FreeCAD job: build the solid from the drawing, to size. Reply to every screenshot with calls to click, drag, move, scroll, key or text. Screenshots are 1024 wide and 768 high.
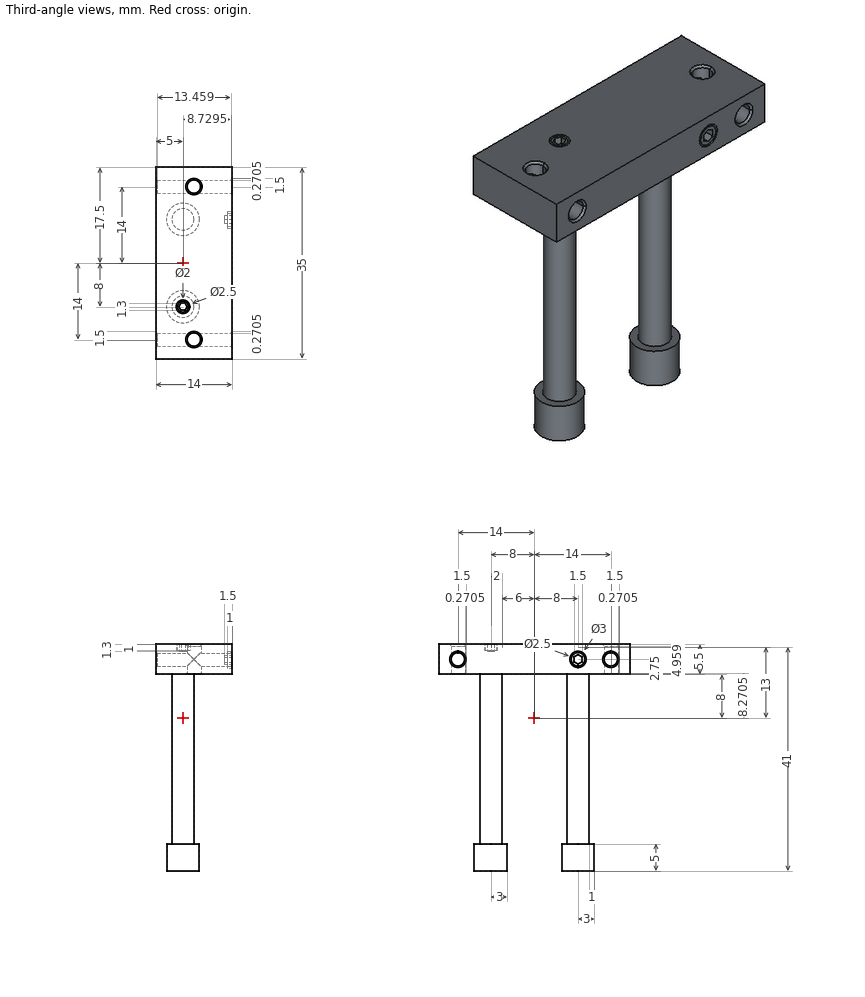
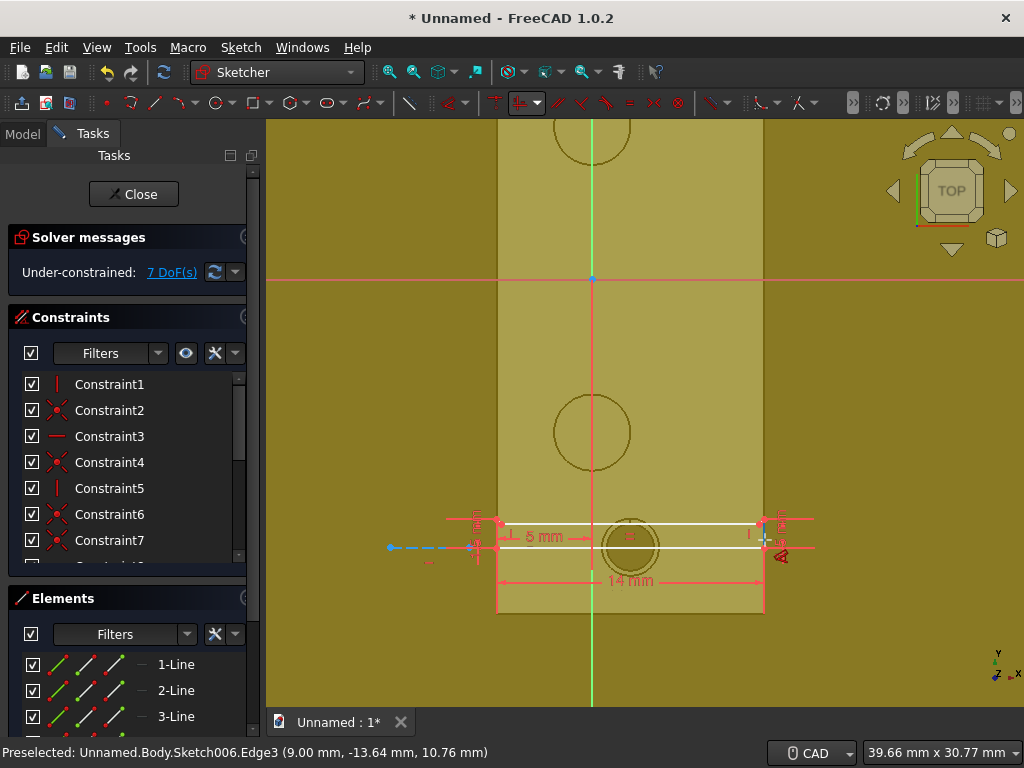
click(497, 548)
click(463, 414)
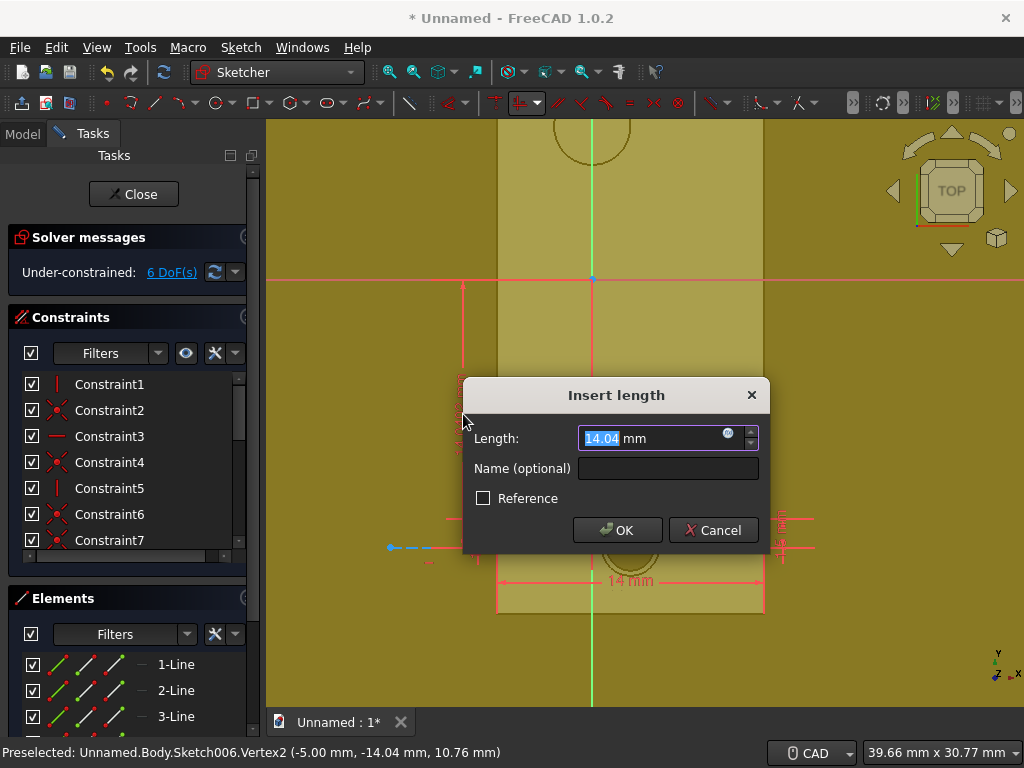
text(14)
key(Return)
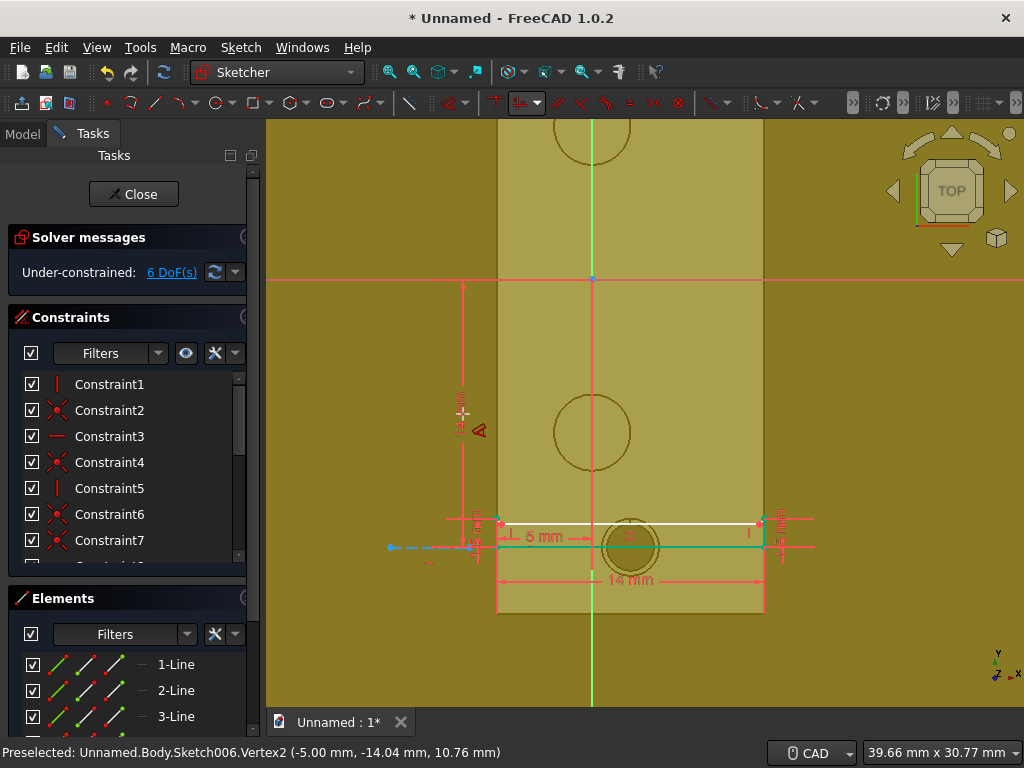
click(470, 548)
click(436, 352)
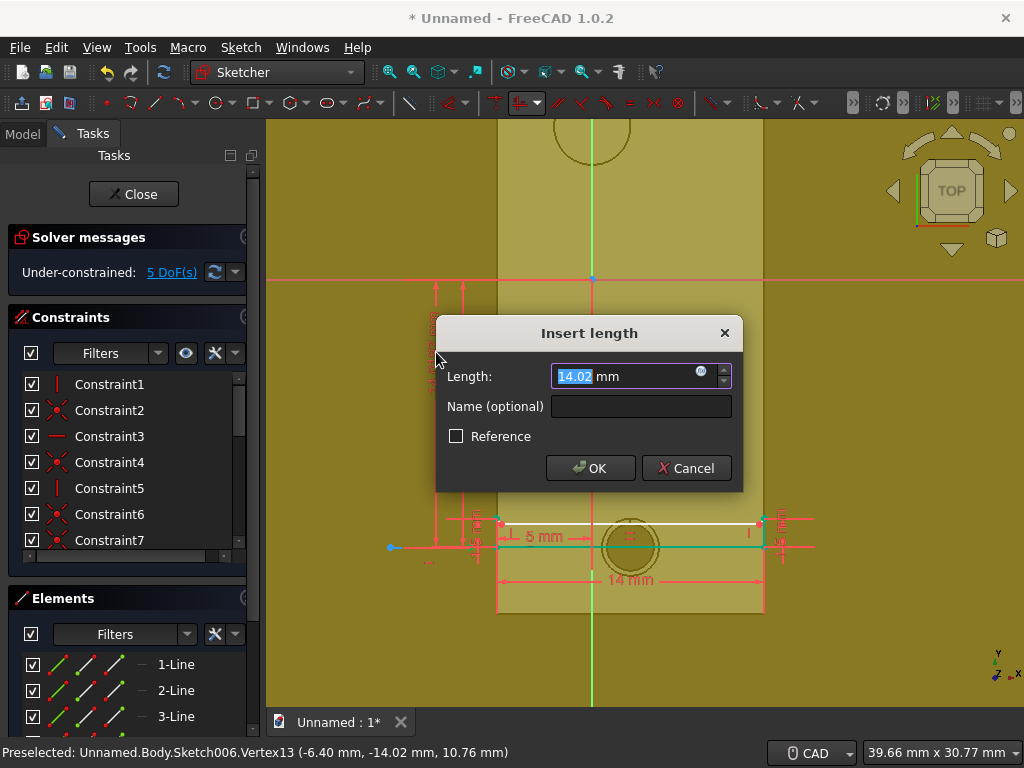
text(14)
key(Return)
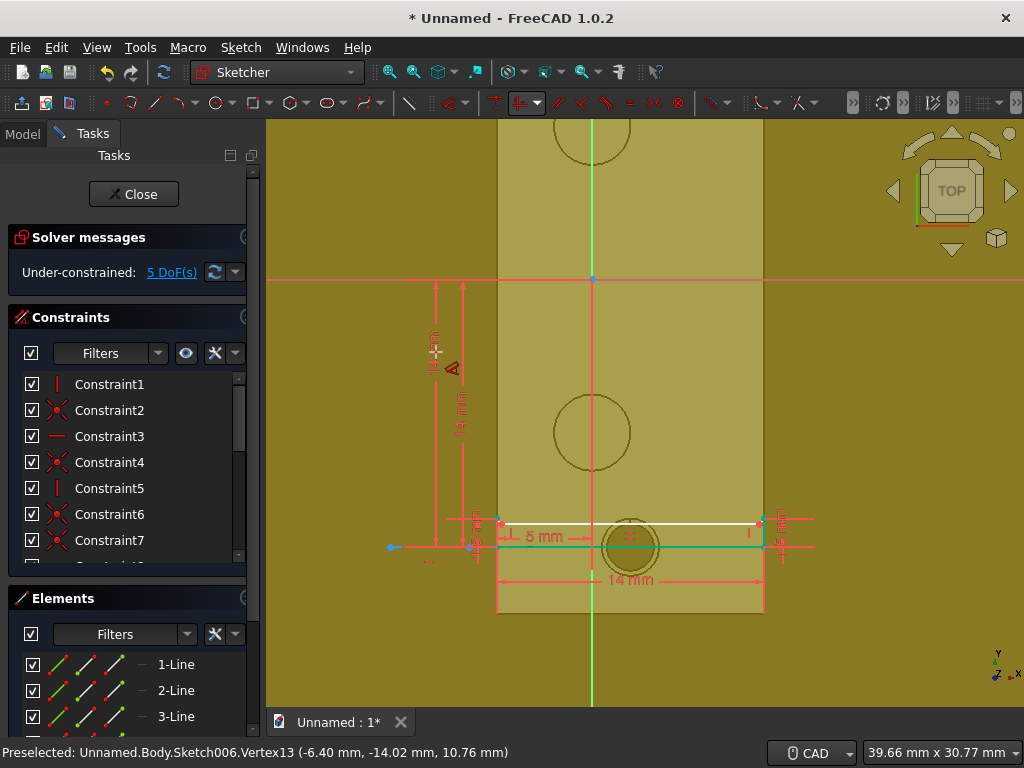
click(682, 524)
click(631, 490)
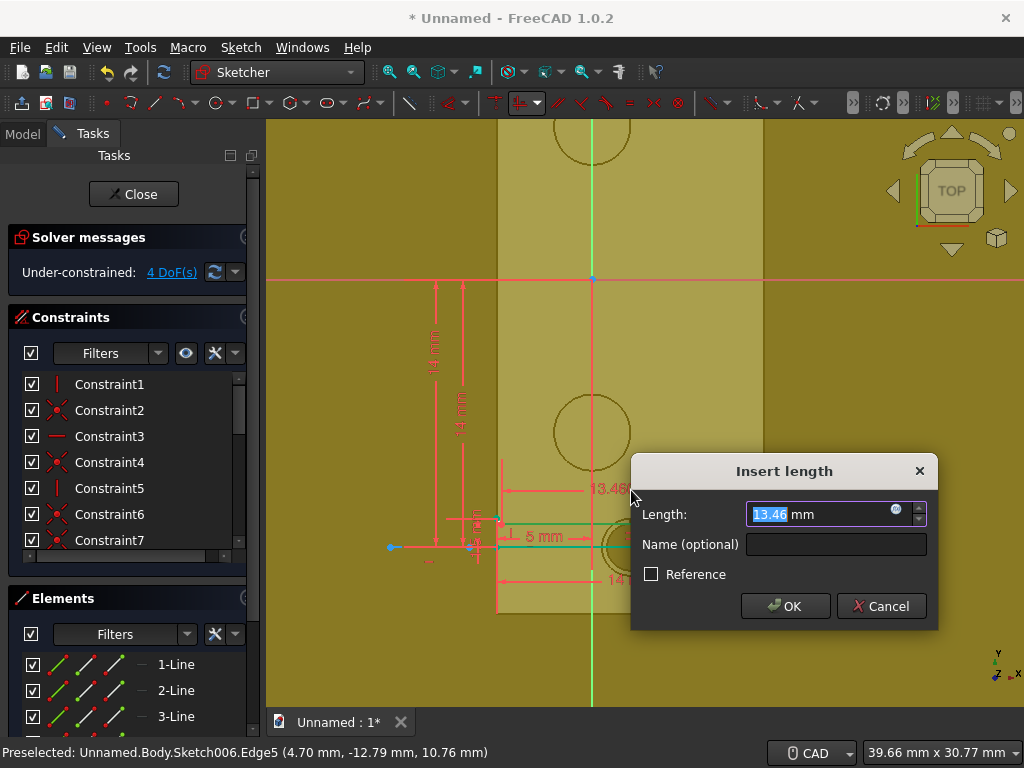
text(13.459)
key(Return)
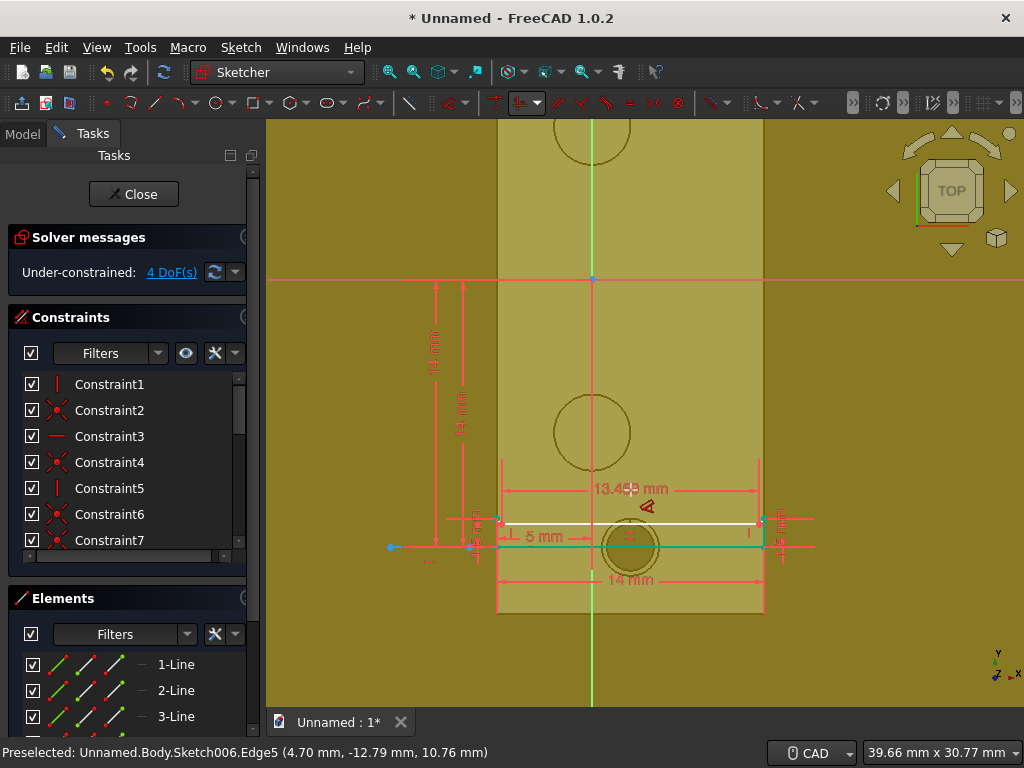
scroll(759, 524, up, 3)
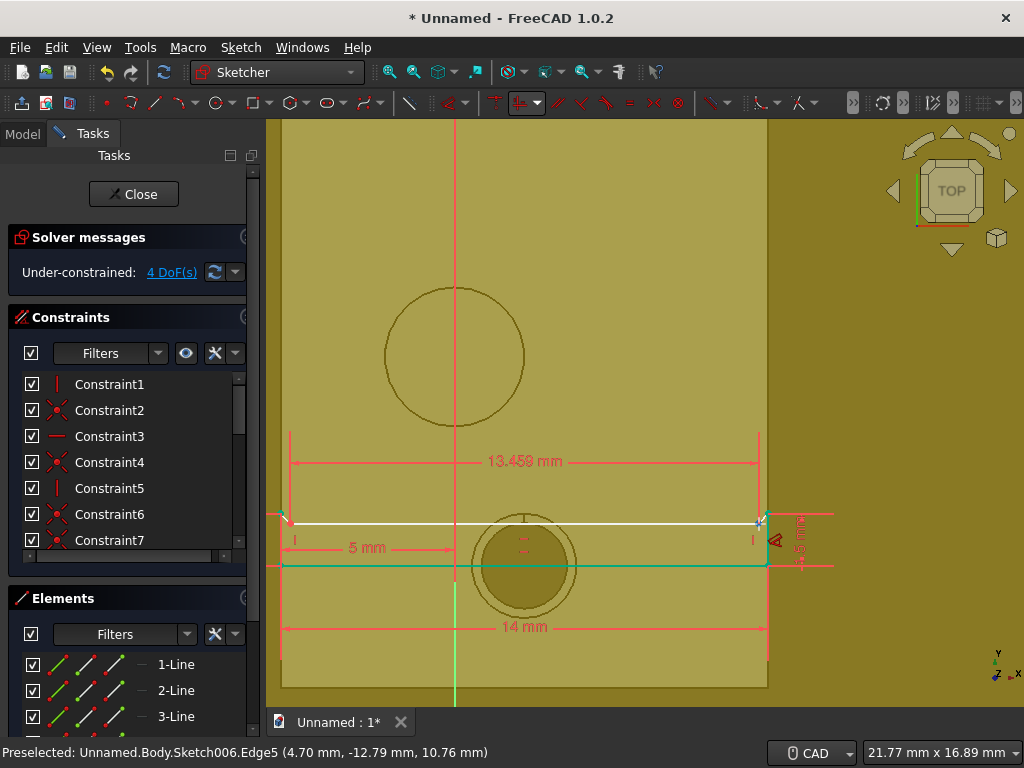
click(759, 524)
click(607, 582)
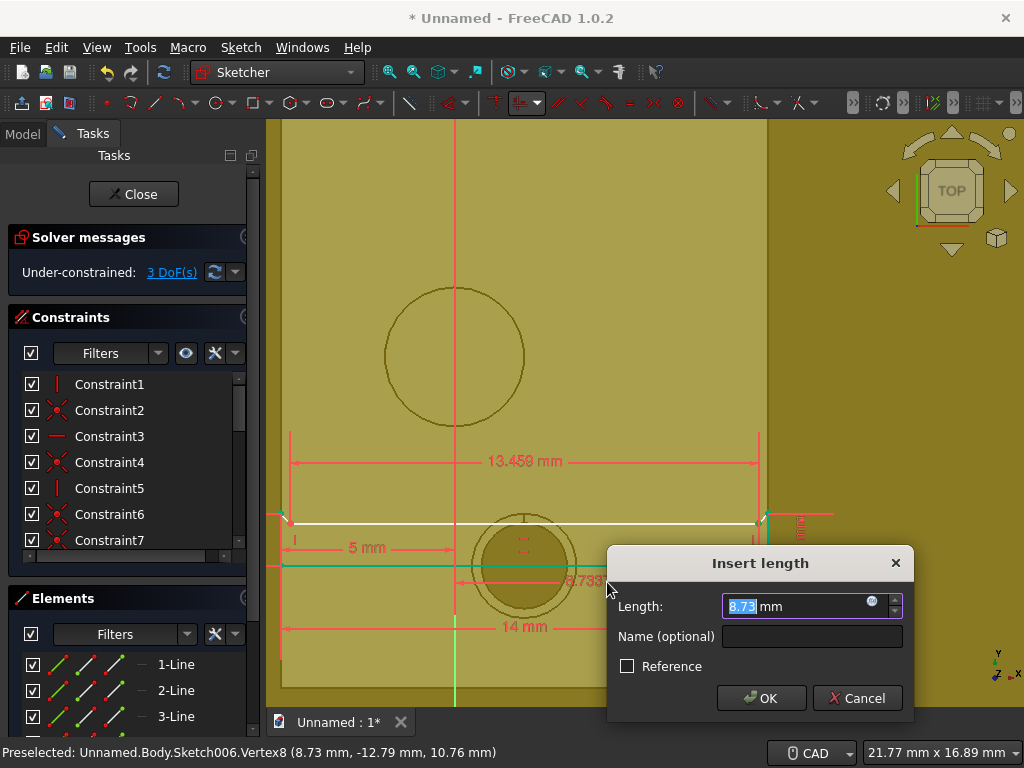
text(8.7295)
key(Return)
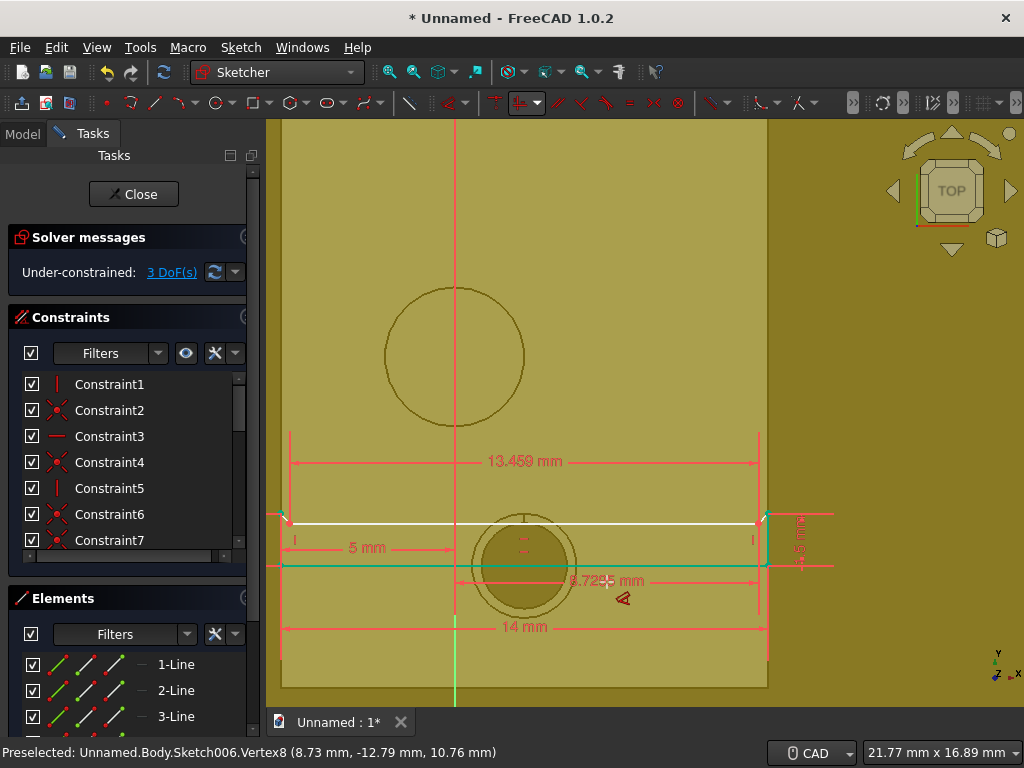
scroll(762, 520, up, 8)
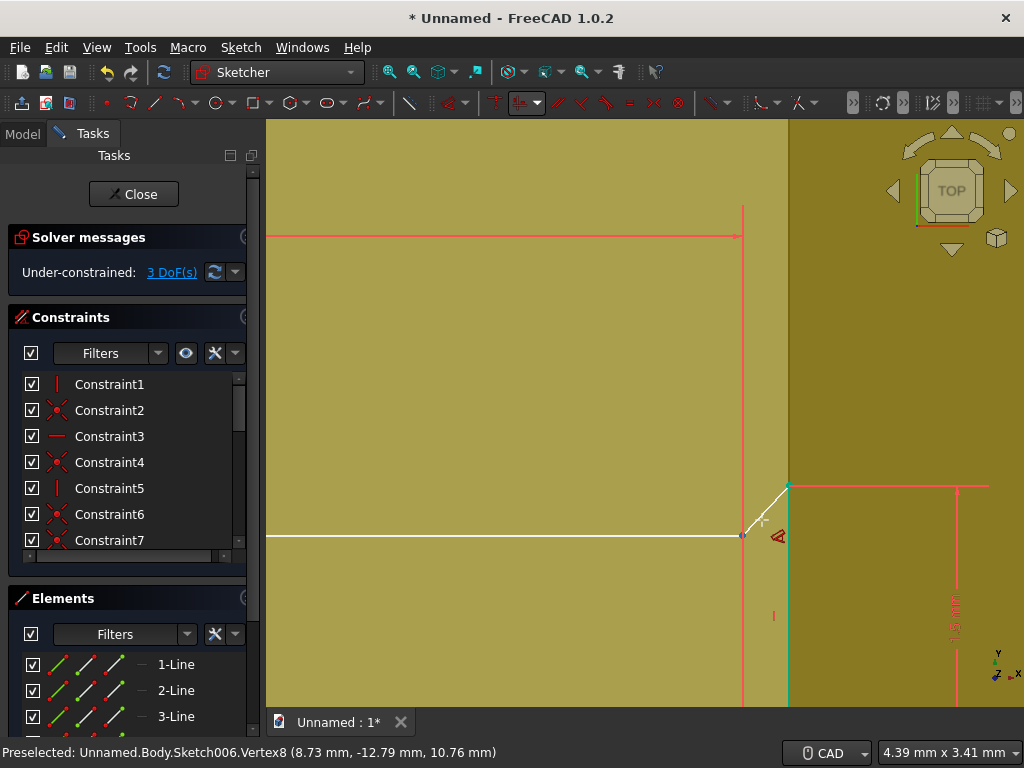
click(761, 516)
click(823, 511)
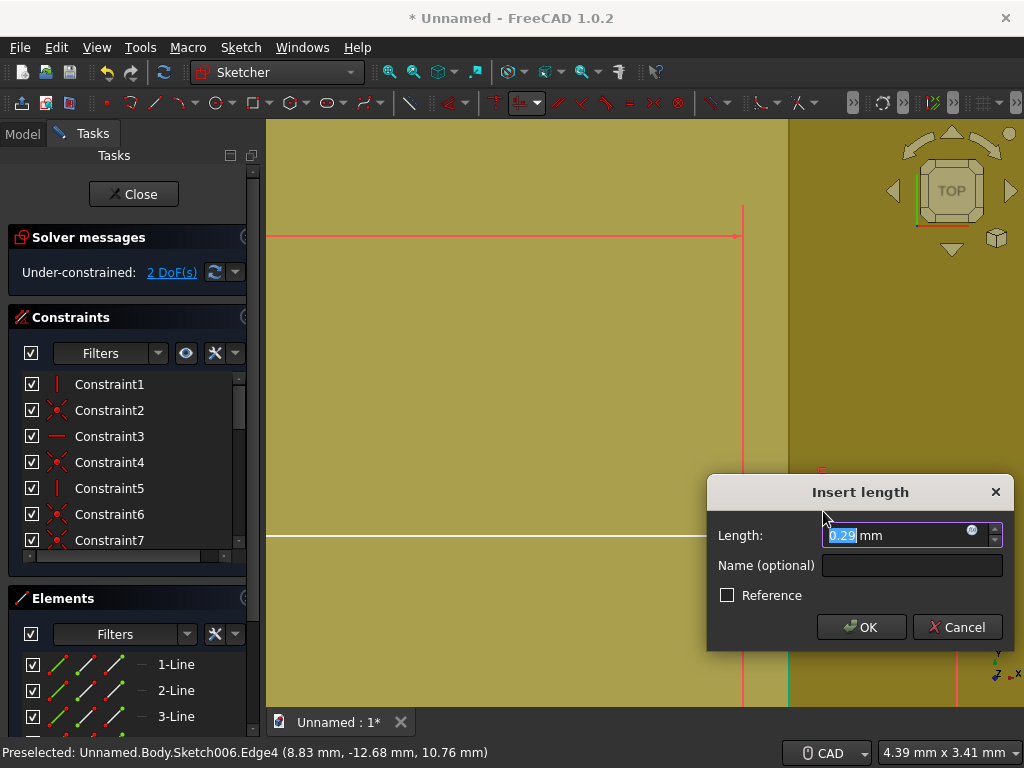
text(0.2705)
key(Return)
key(Escape)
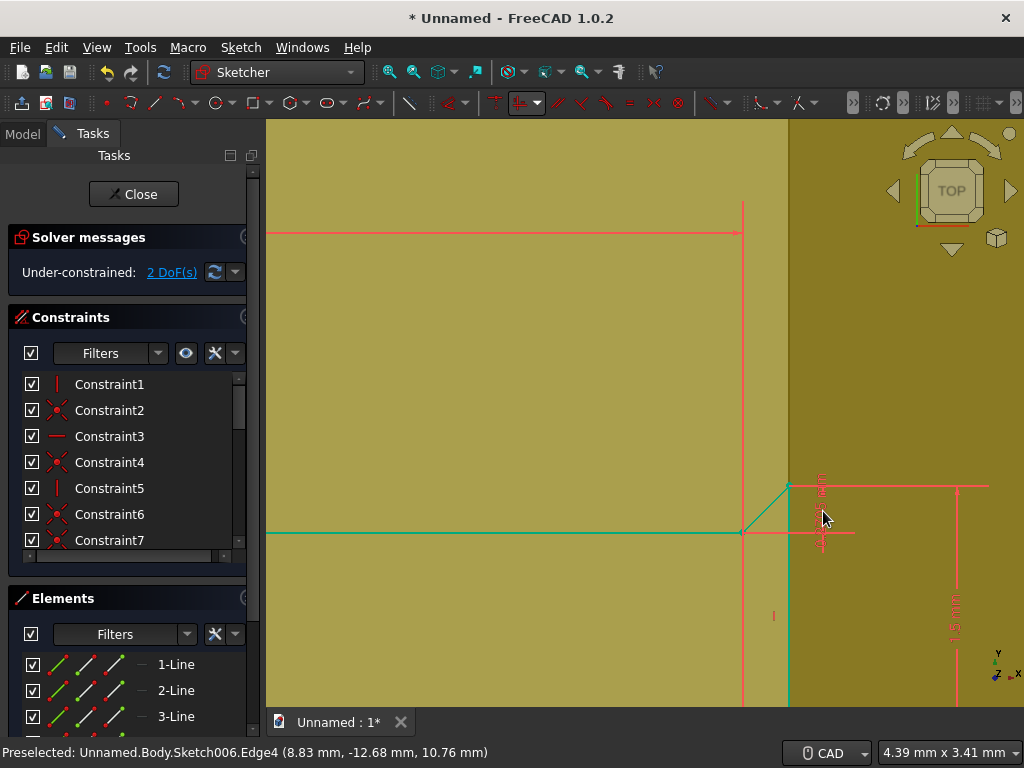
click(134, 194)